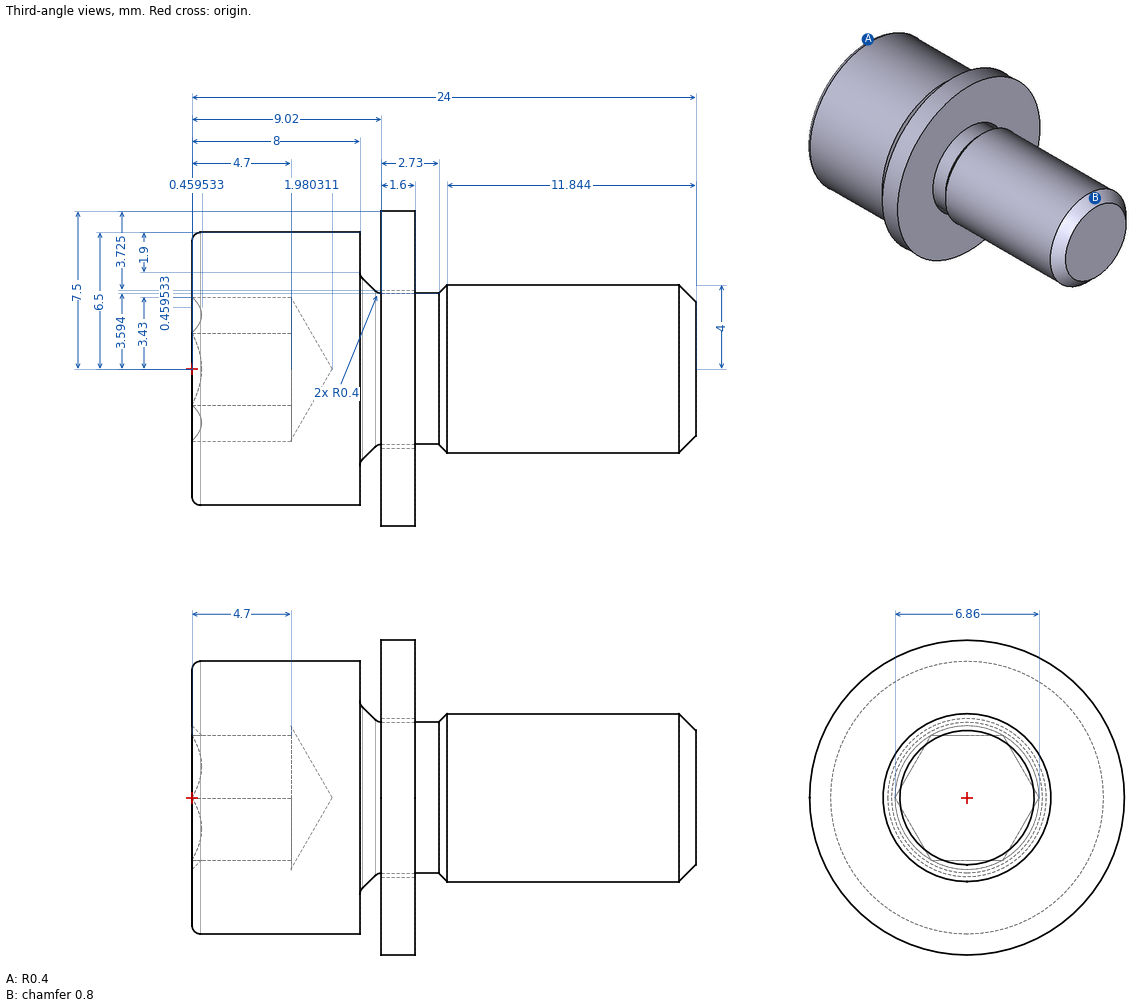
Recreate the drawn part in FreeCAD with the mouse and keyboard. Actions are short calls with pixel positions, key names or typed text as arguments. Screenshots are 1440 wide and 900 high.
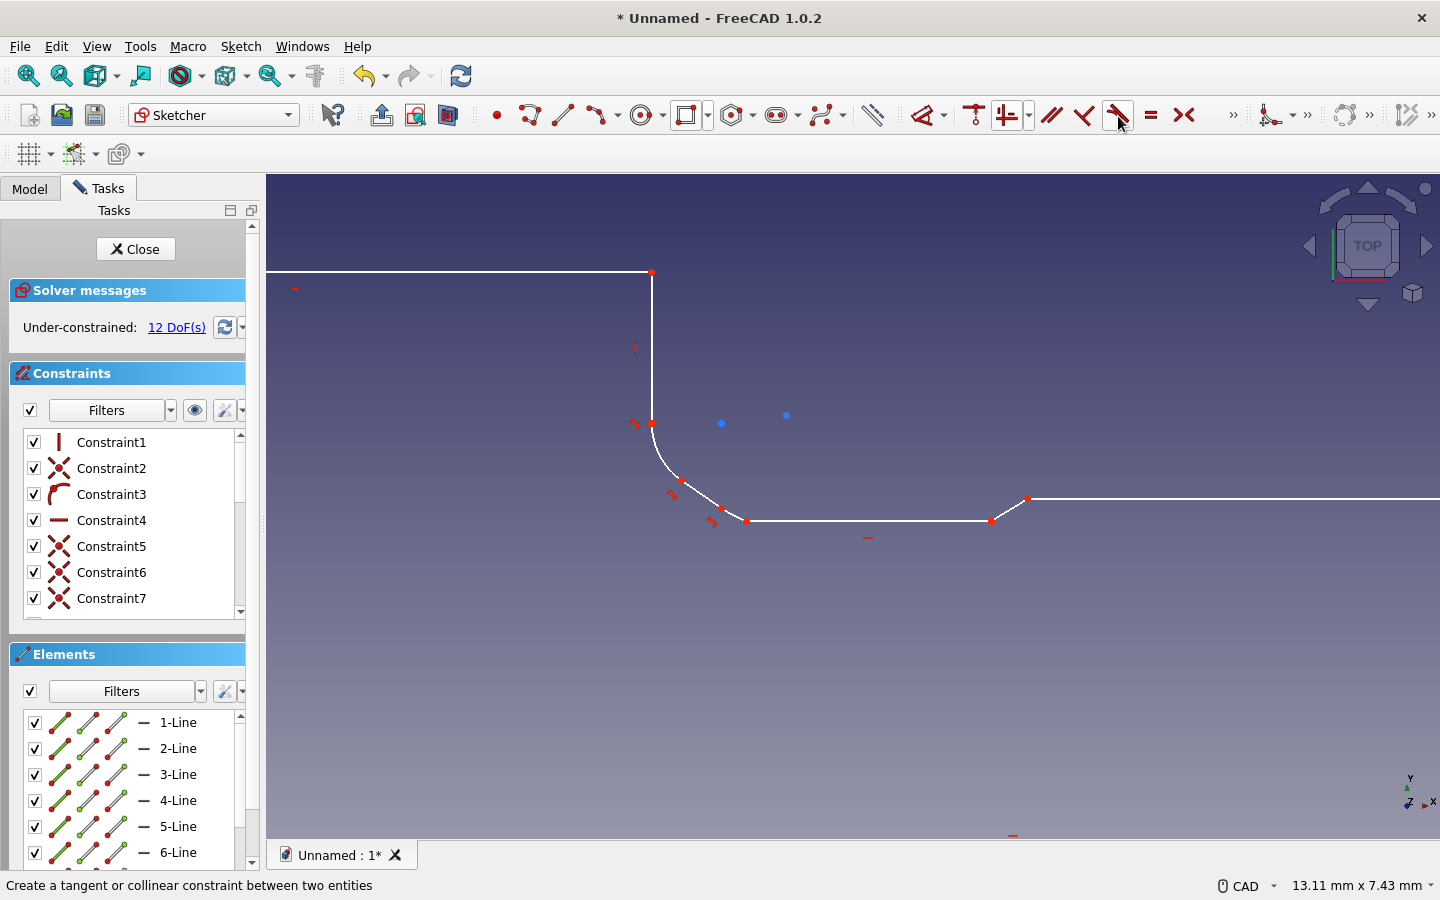
click(918, 521)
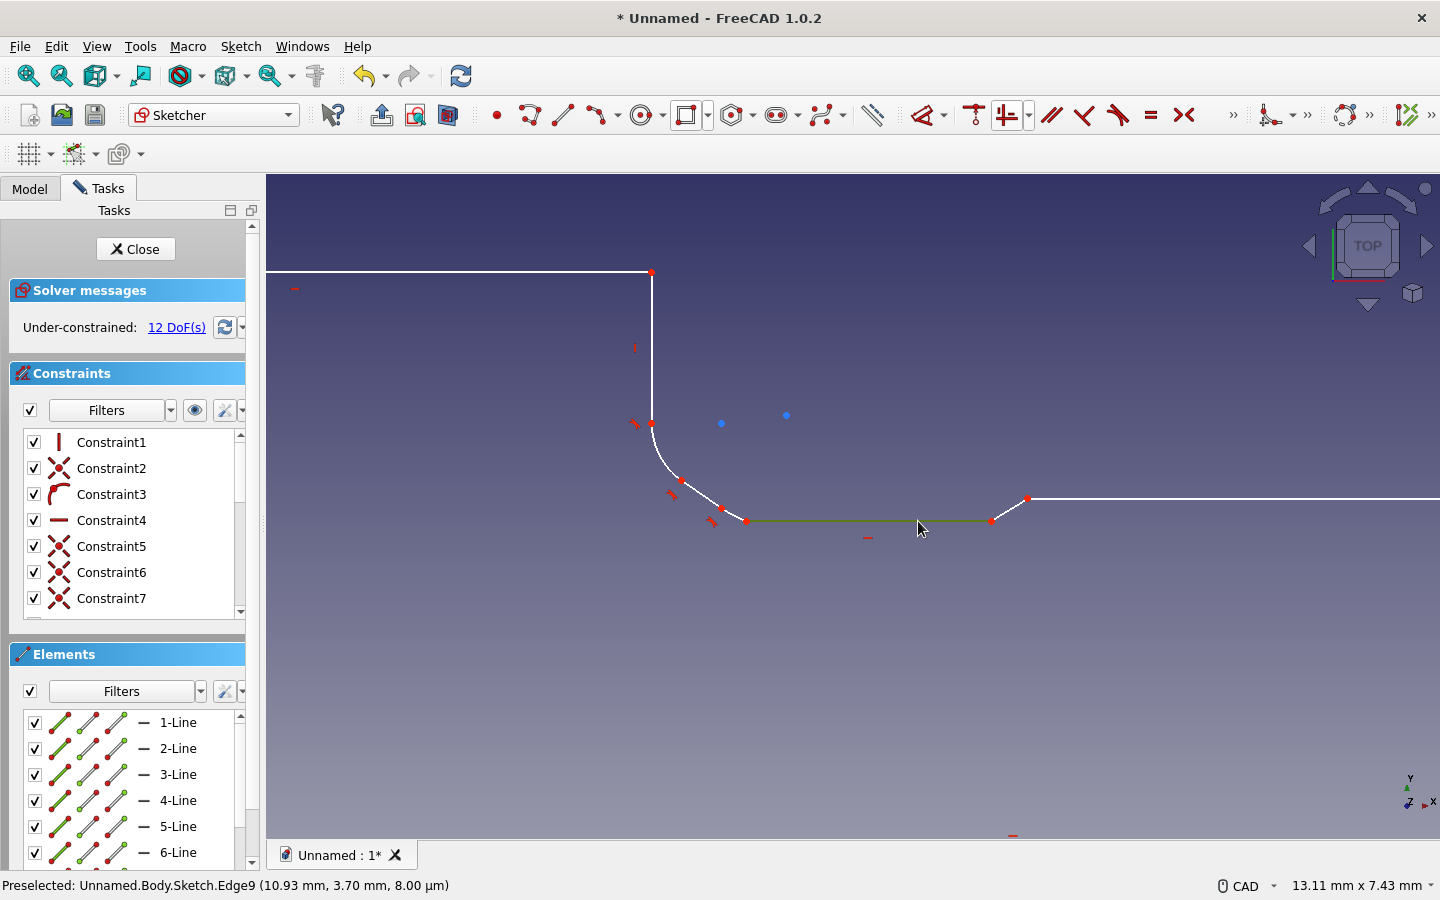
click(734, 516)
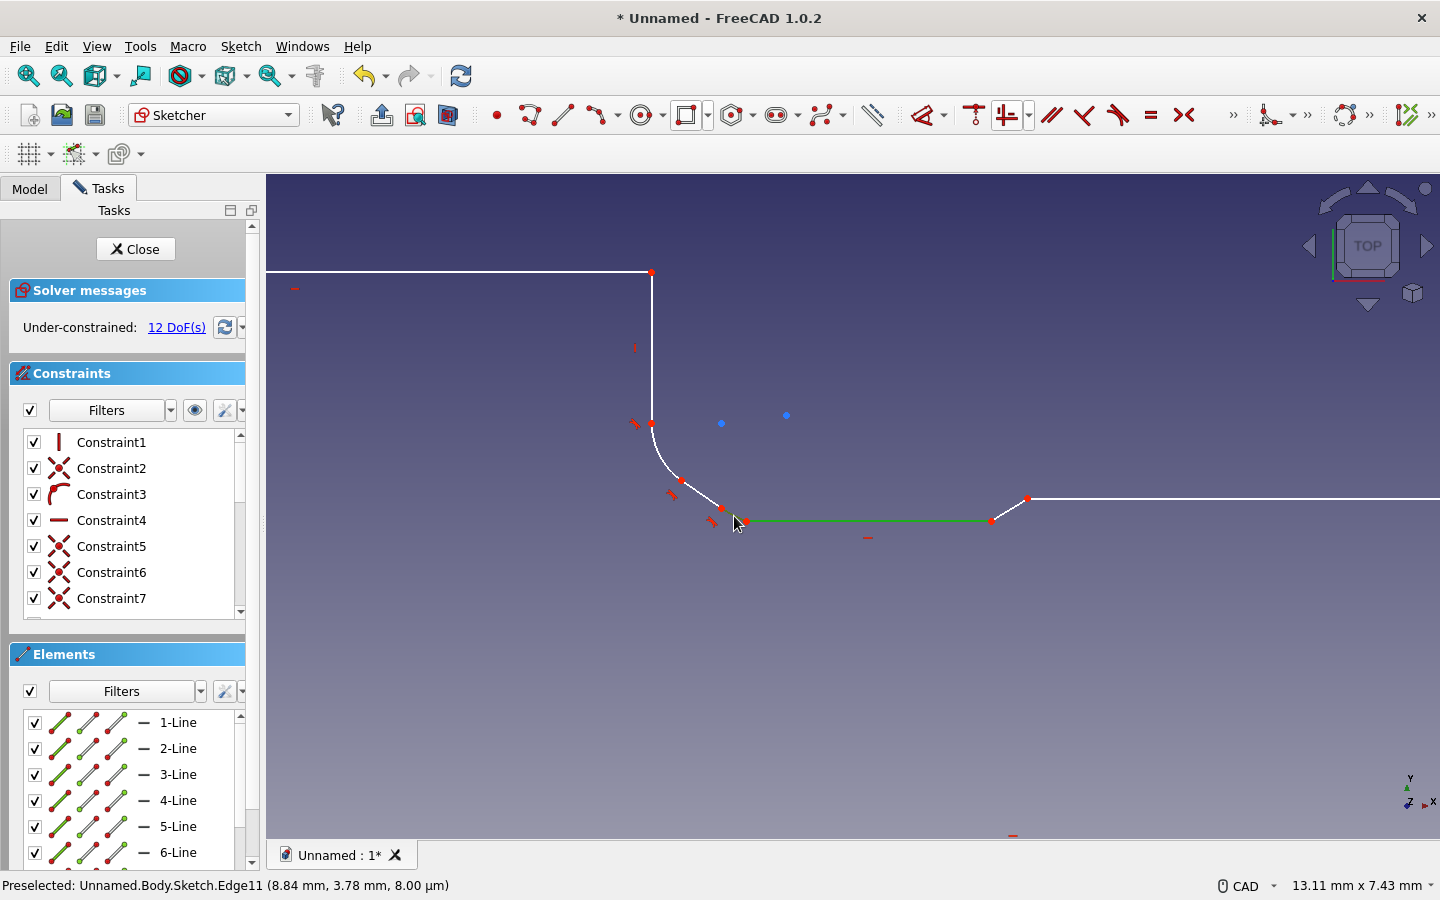
click(1118, 116)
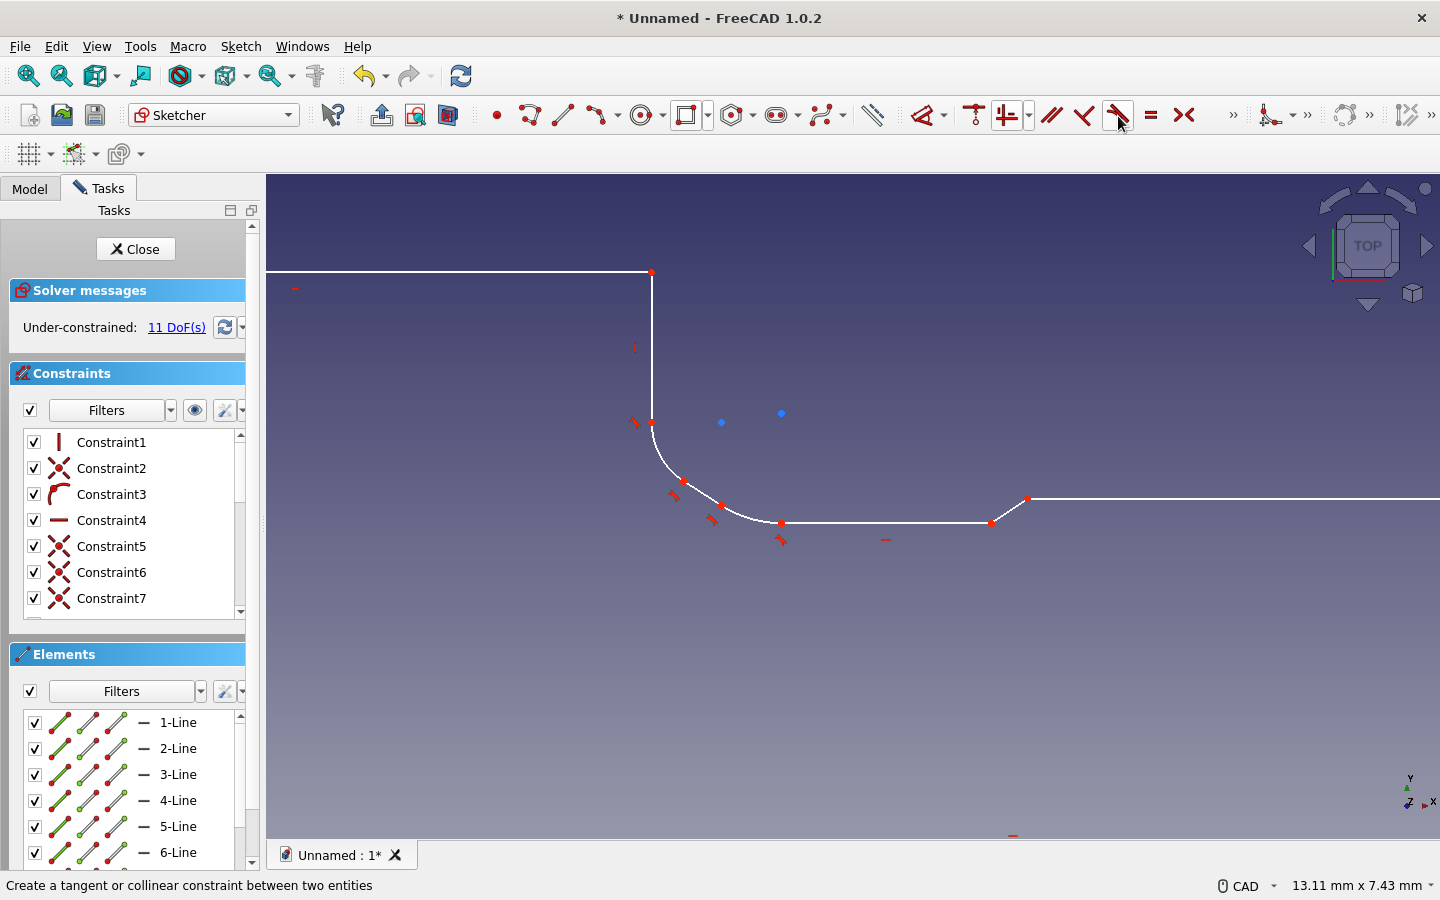
click(655, 443)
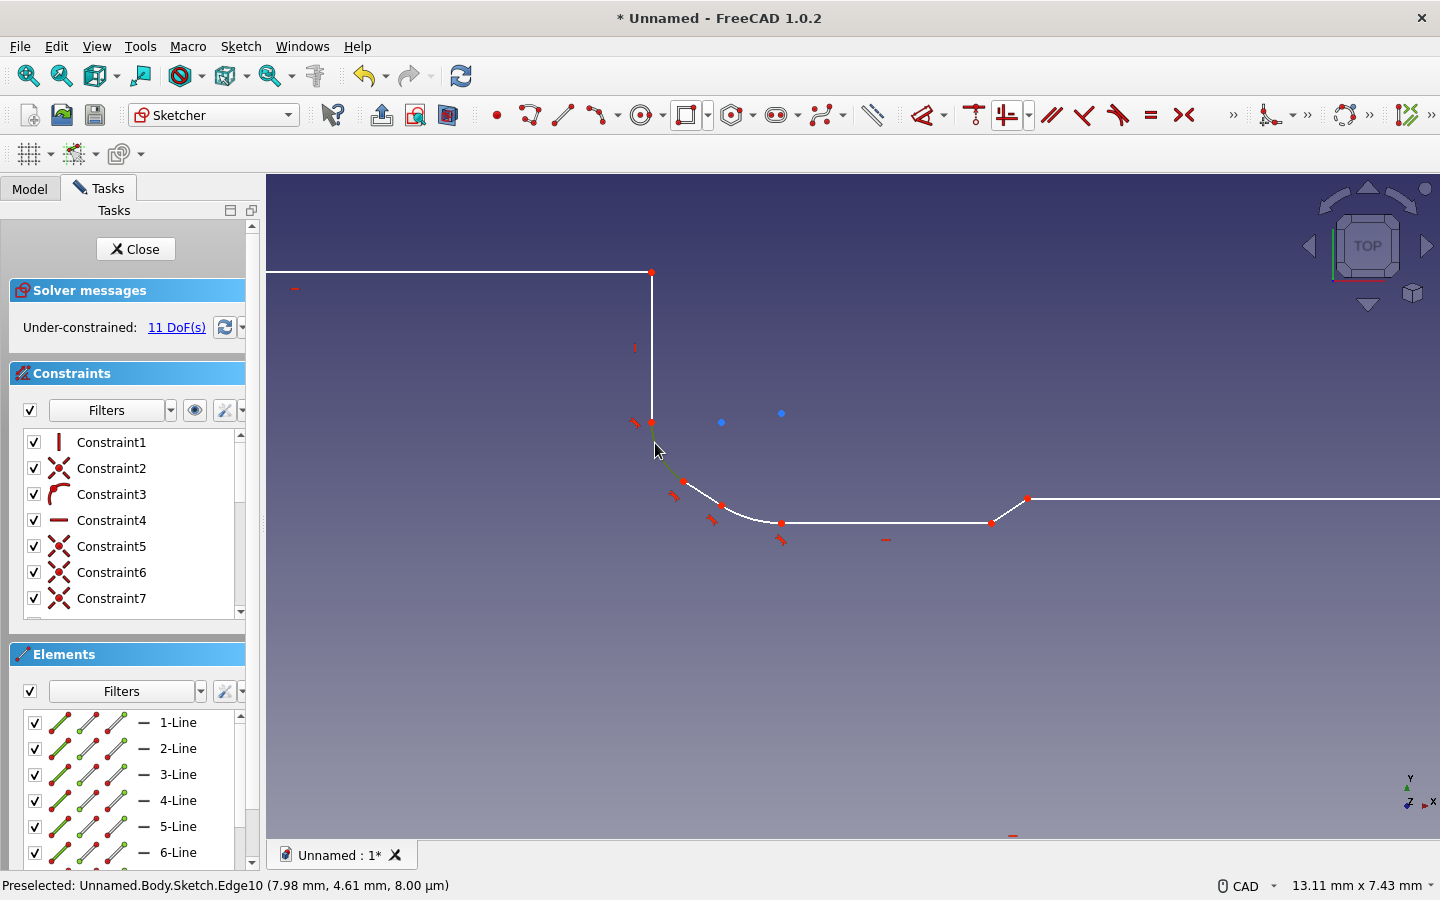
click(738, 514)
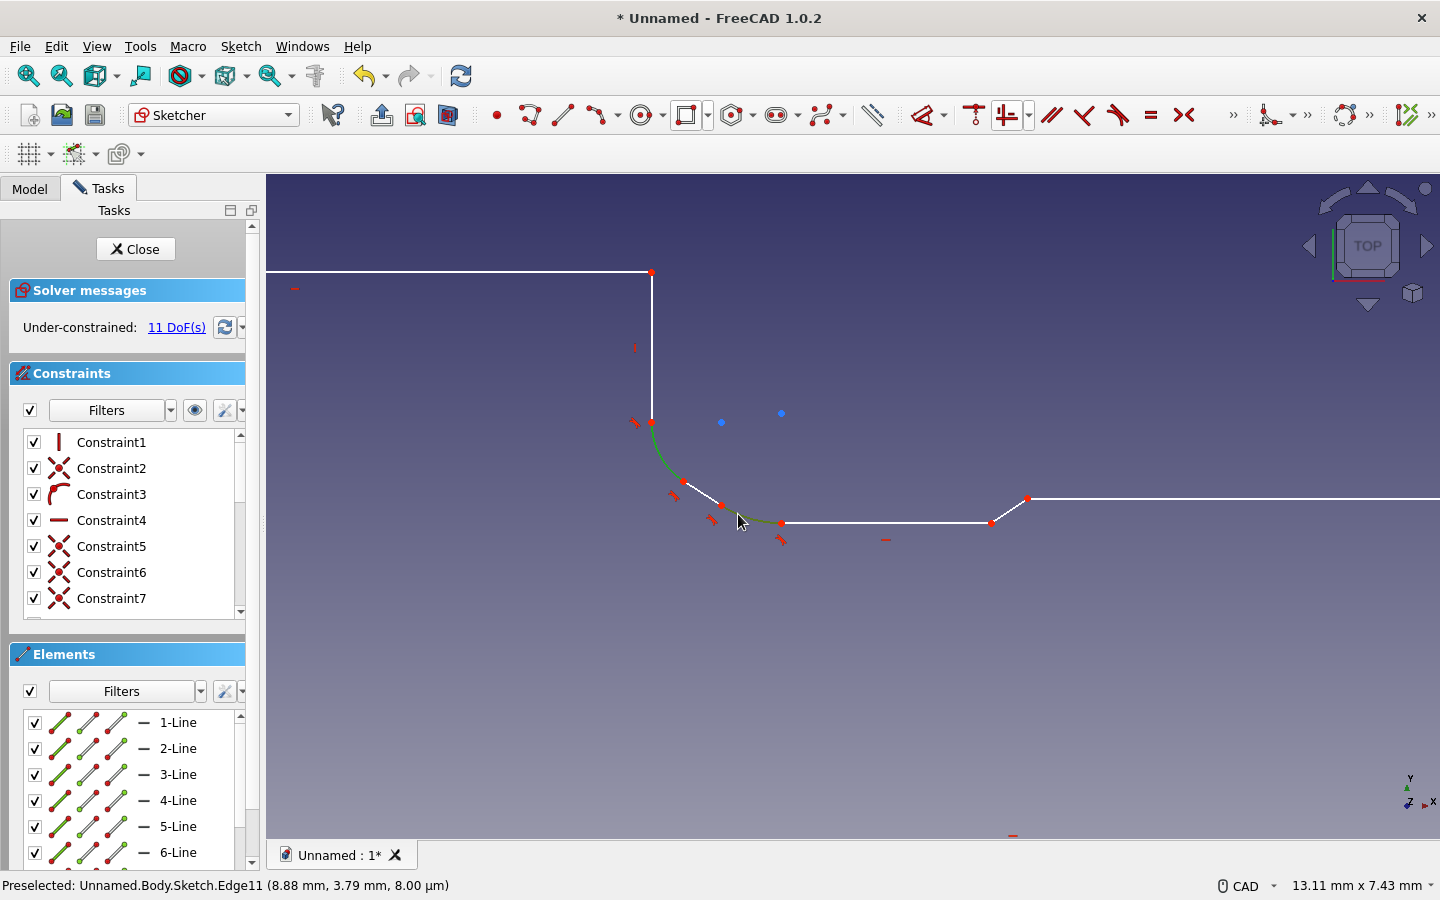
click(1151, 116)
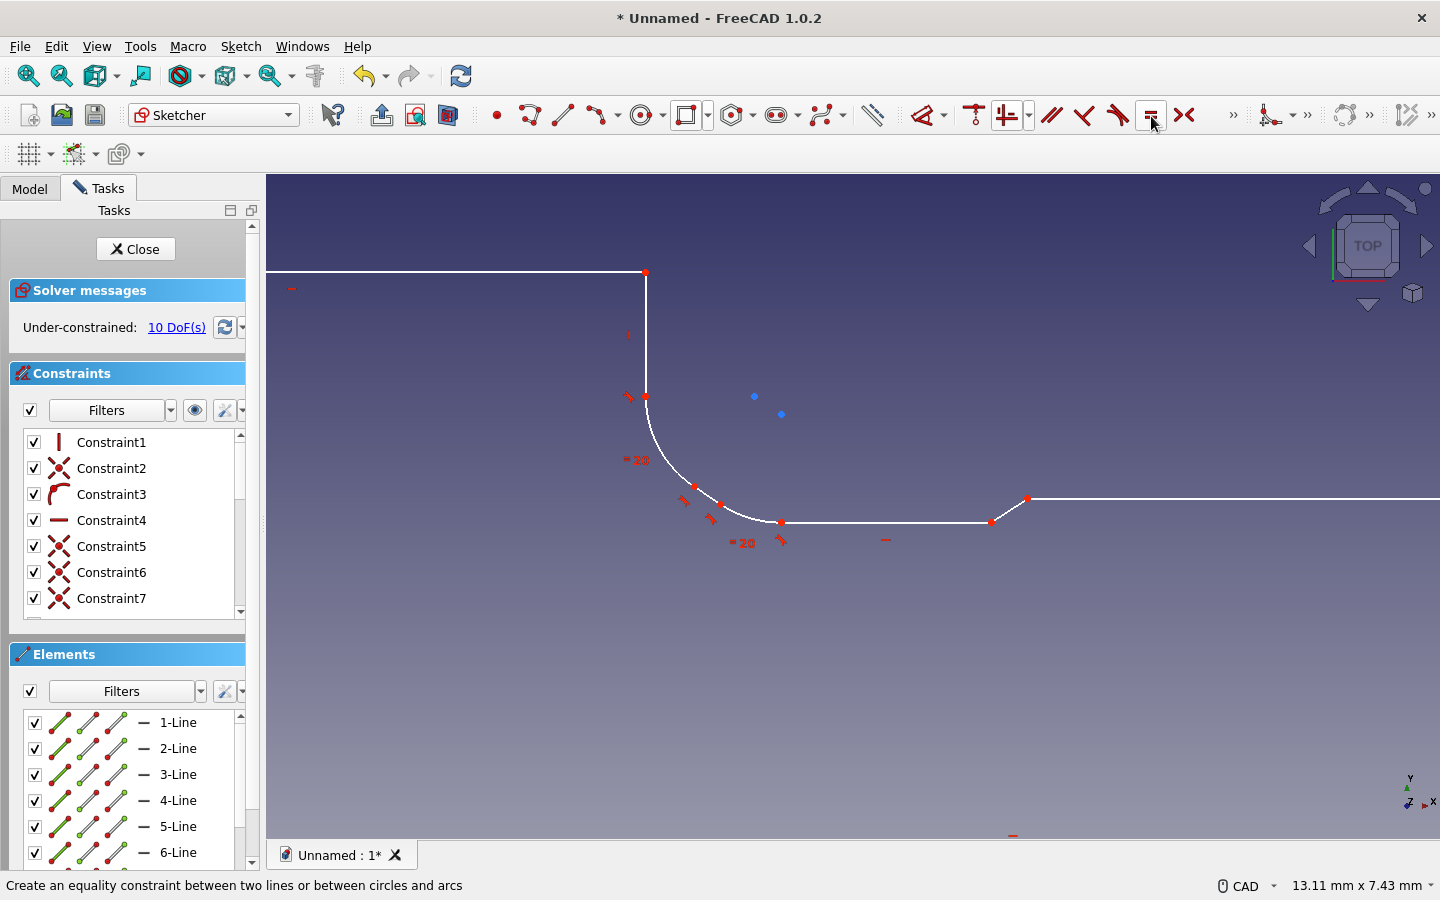
click(922, 116)